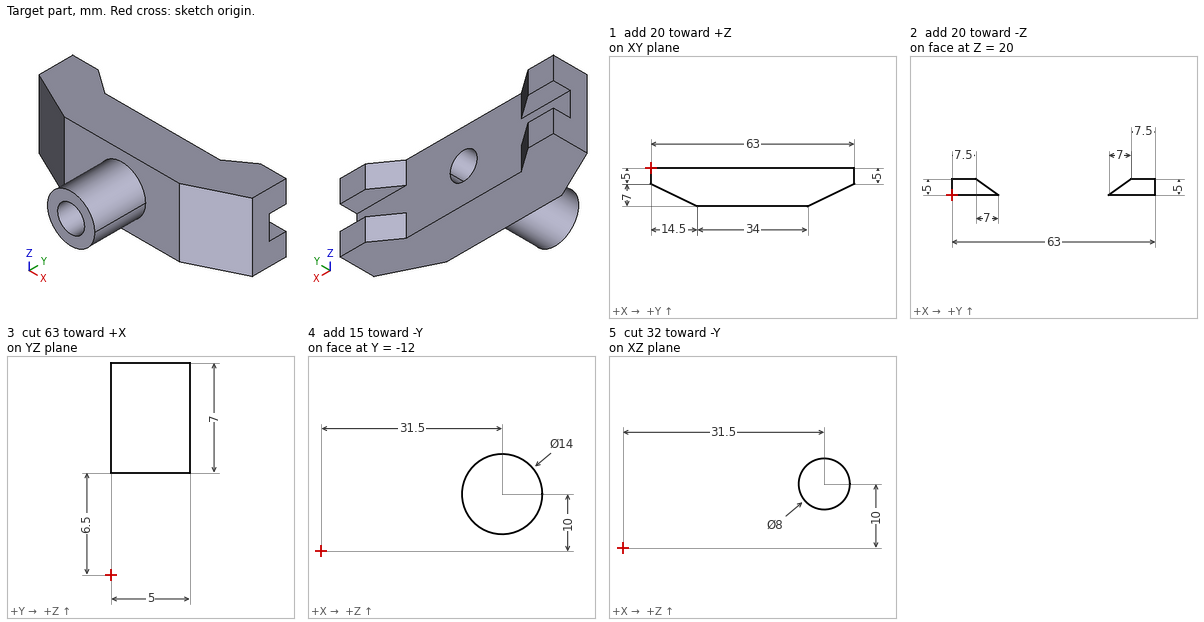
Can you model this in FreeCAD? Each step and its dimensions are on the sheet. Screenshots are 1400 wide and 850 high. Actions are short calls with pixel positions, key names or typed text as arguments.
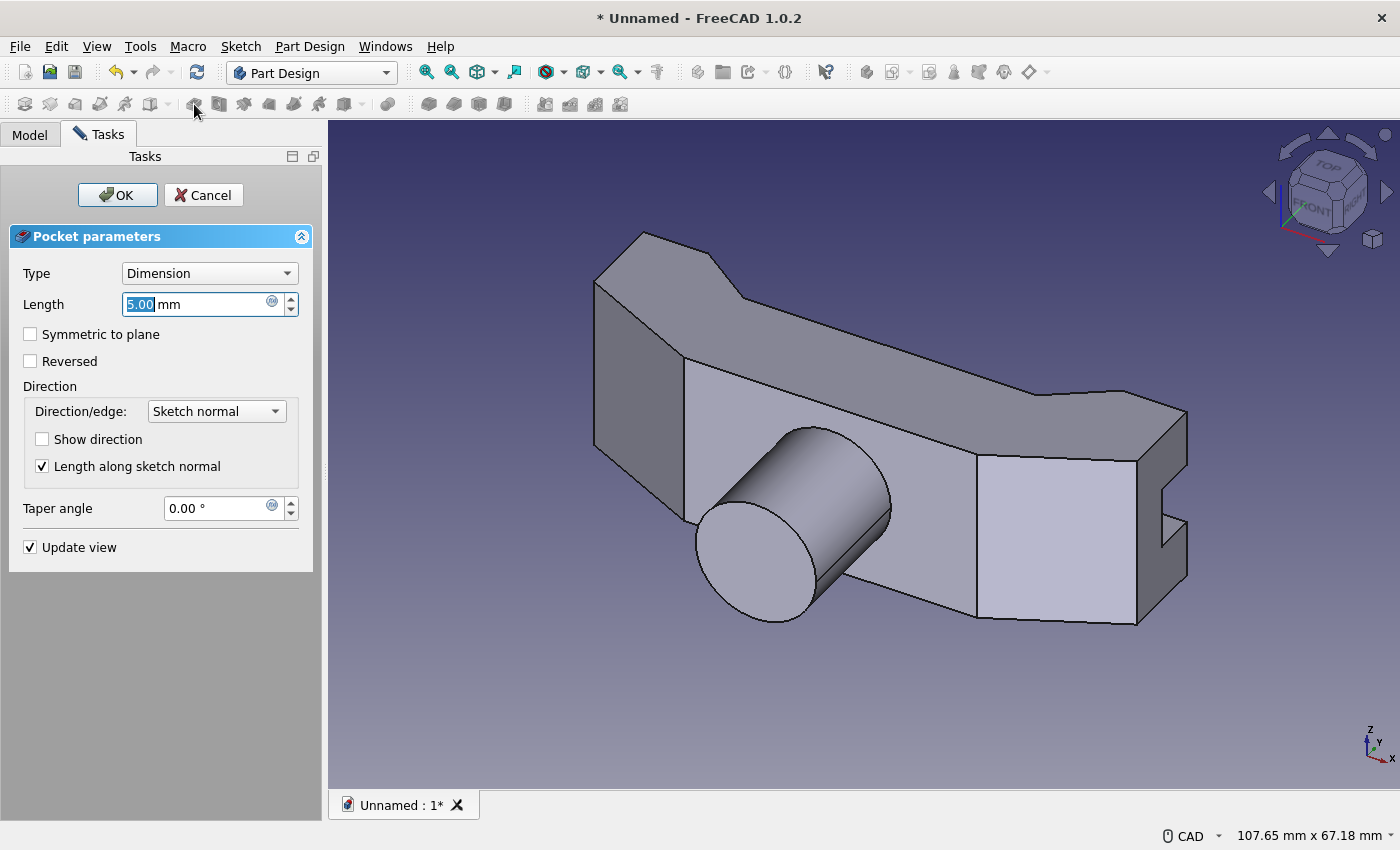
text(32)
key(Tab)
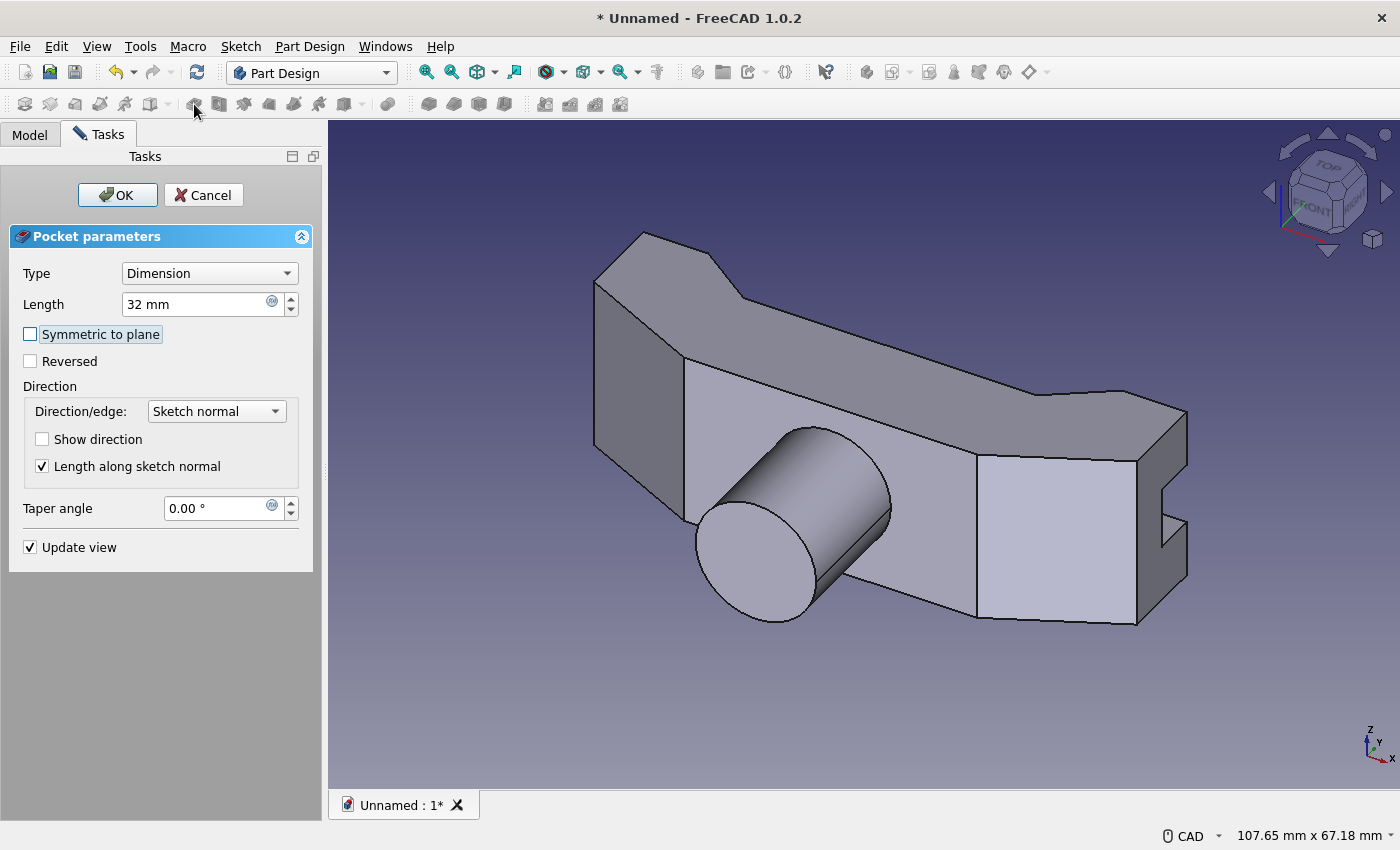
click(31, 361)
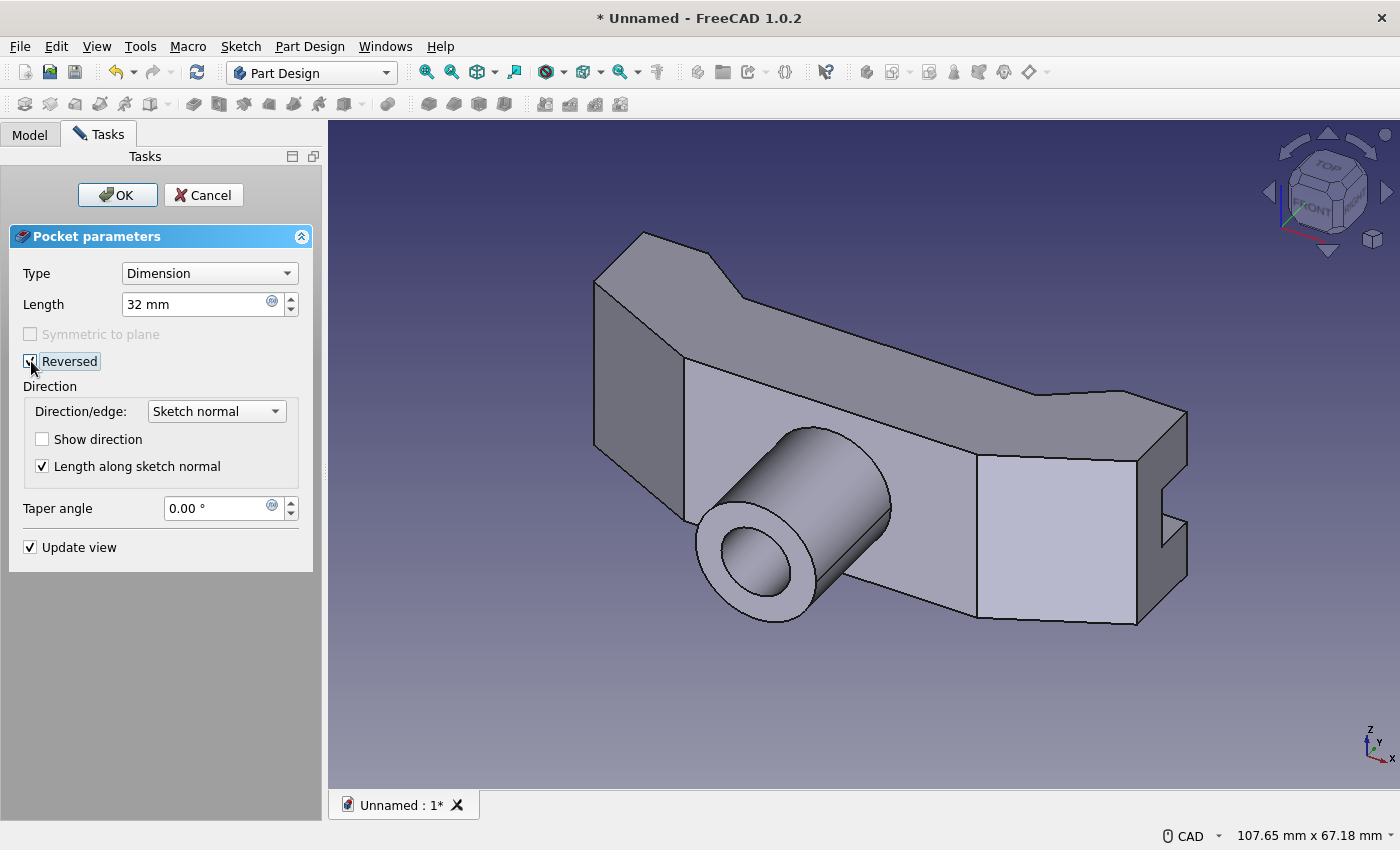
click(118, 195)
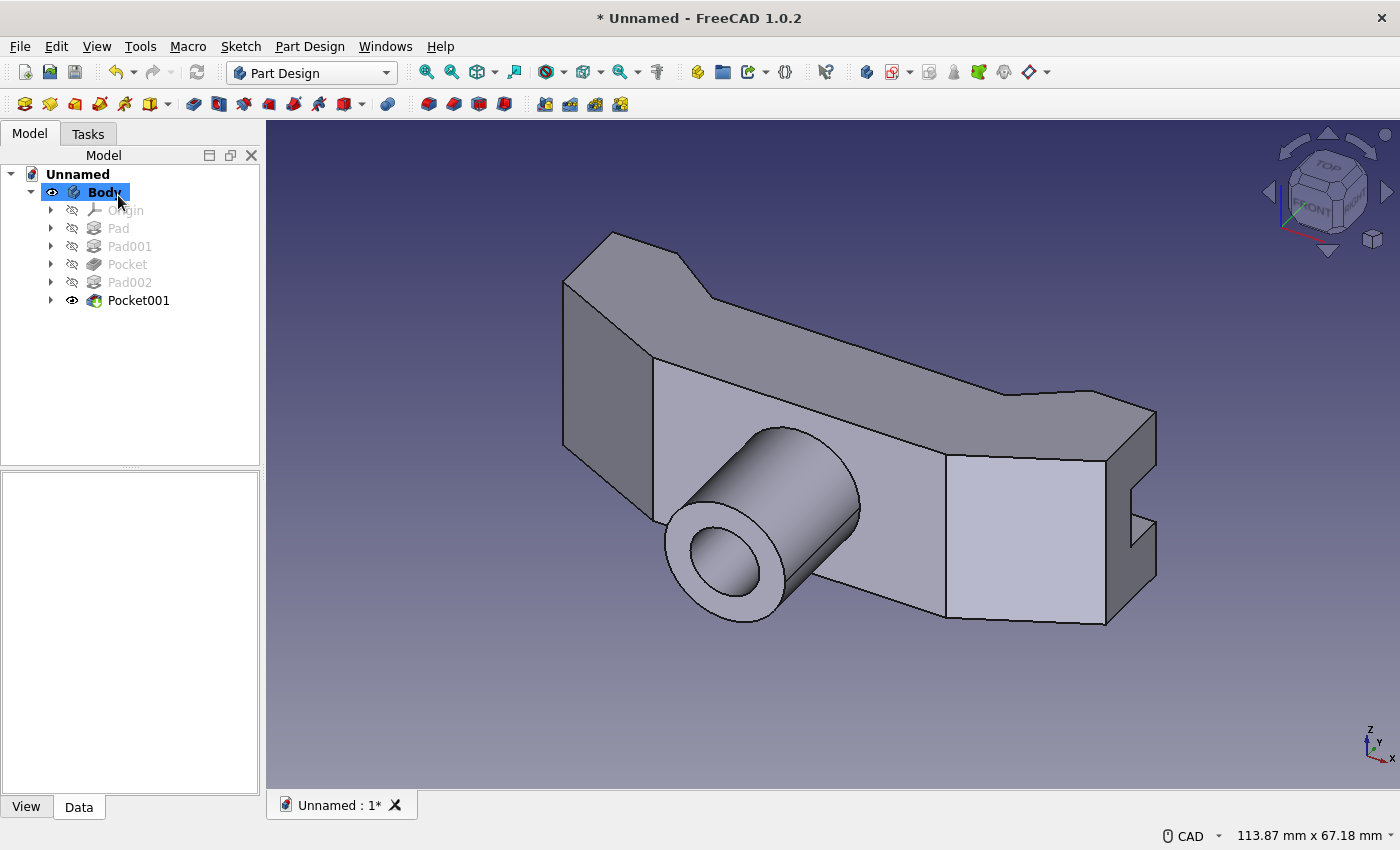
key(0)